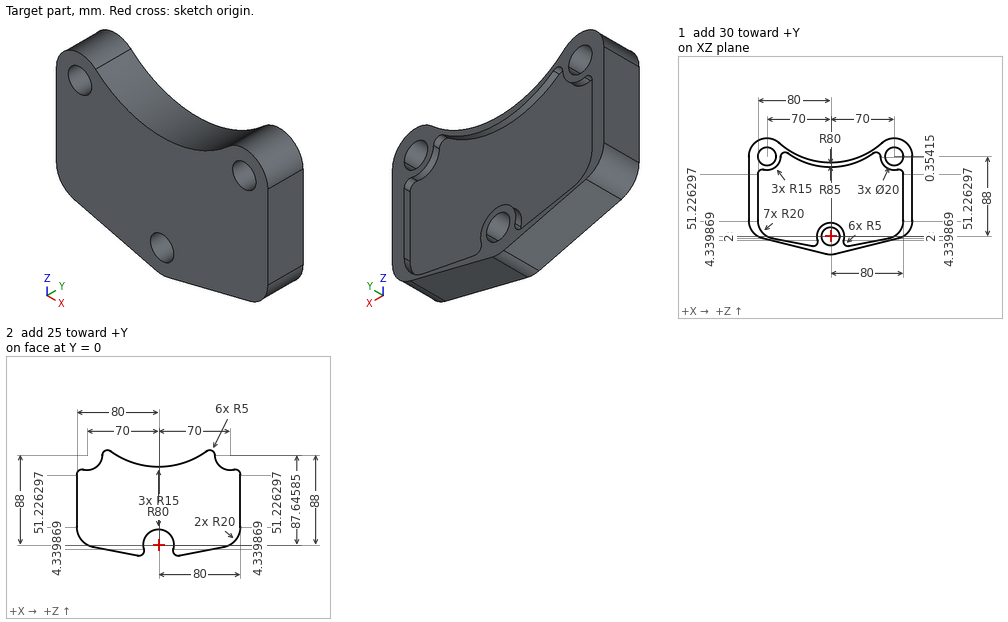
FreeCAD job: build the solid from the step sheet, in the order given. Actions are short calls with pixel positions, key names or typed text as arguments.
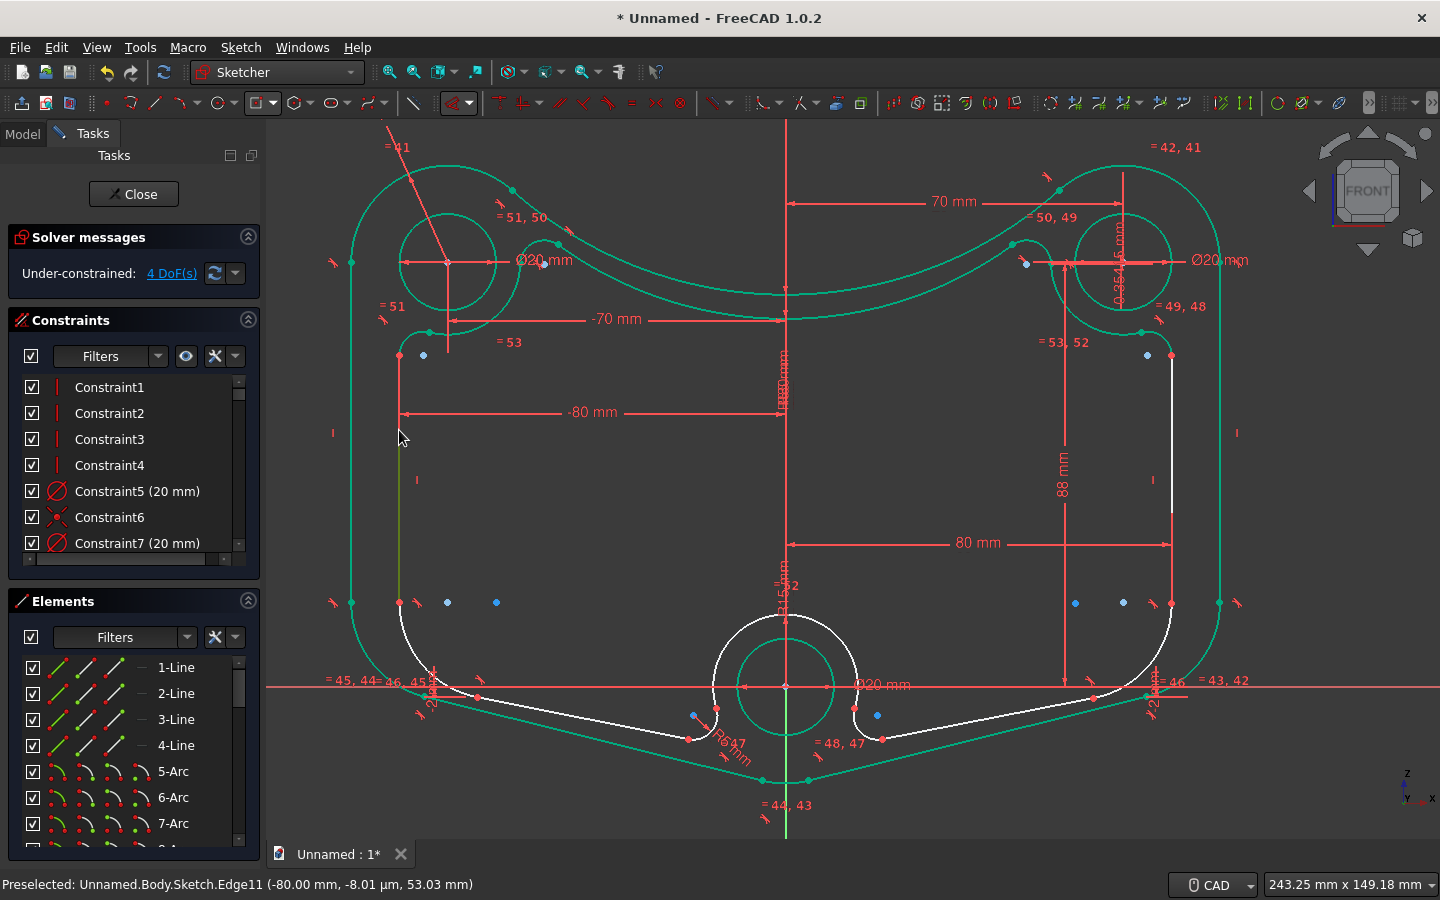
click(472, 104)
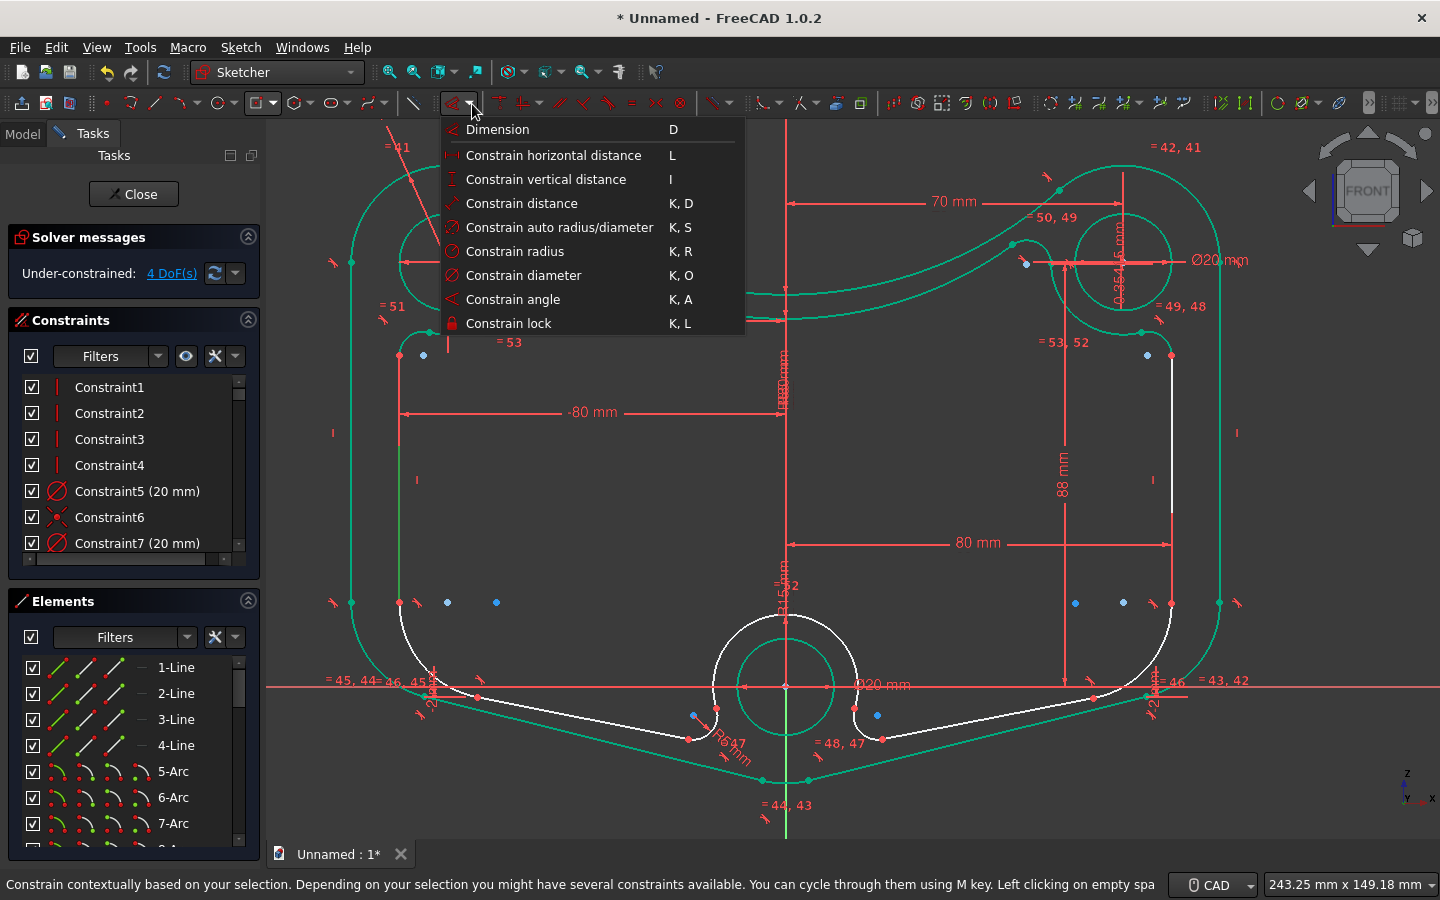
click(593, 179)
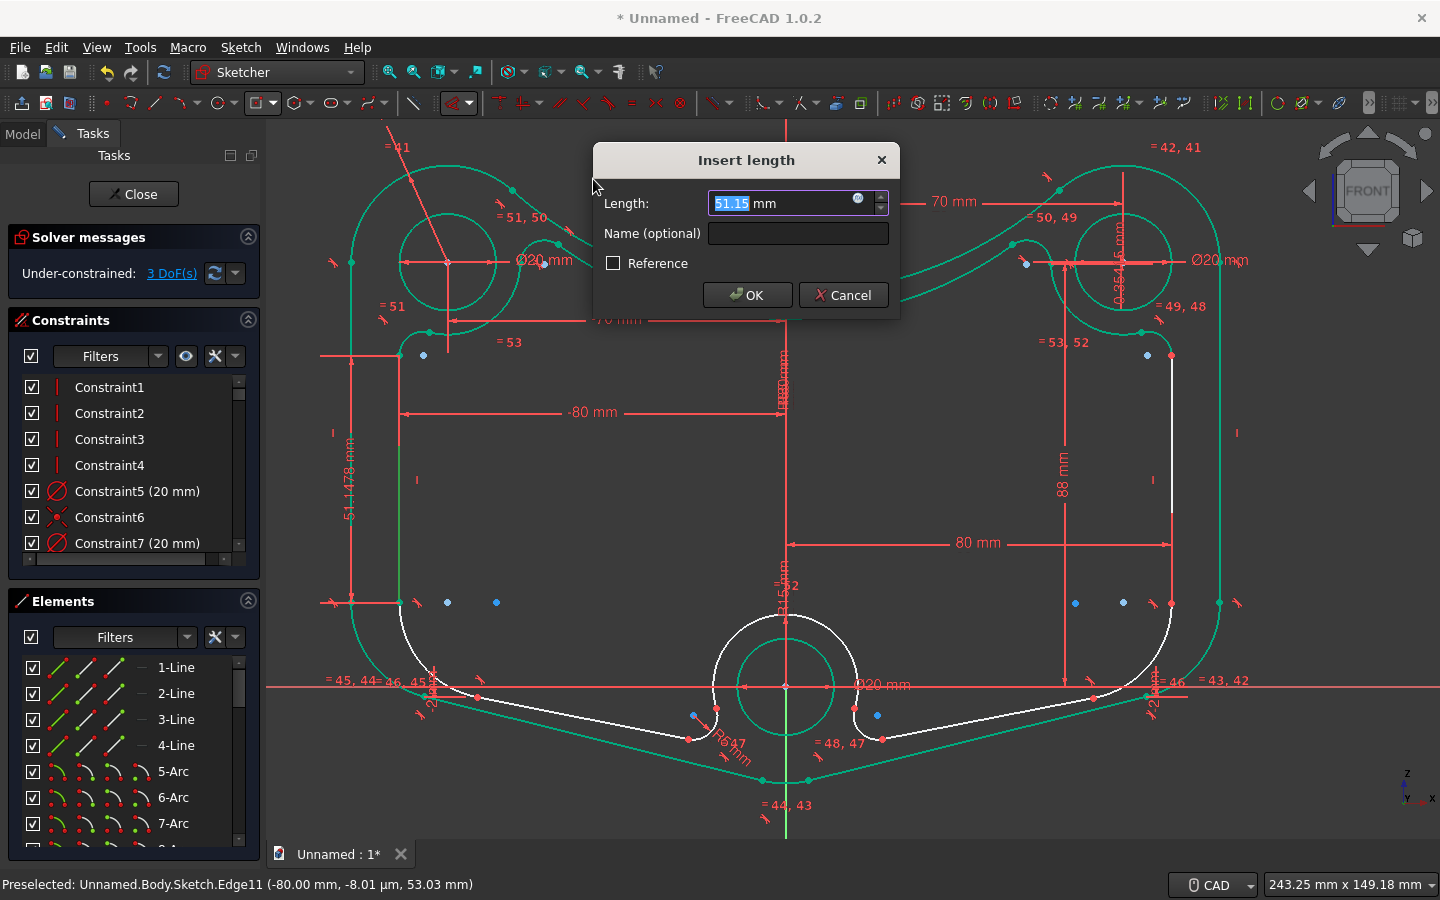
text(51.226297)
key(Return)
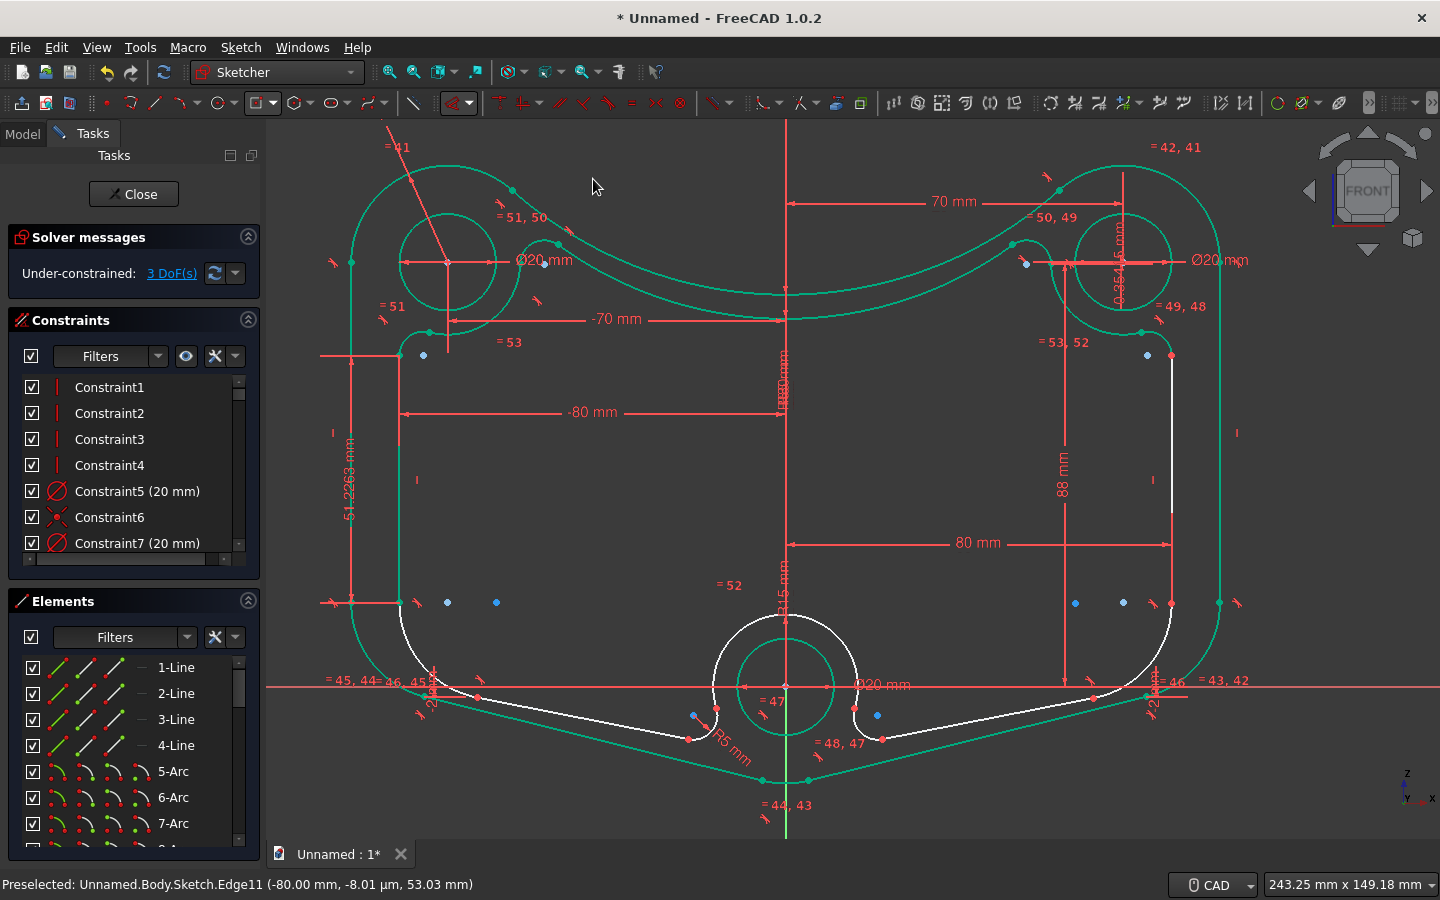
click(1172, 529)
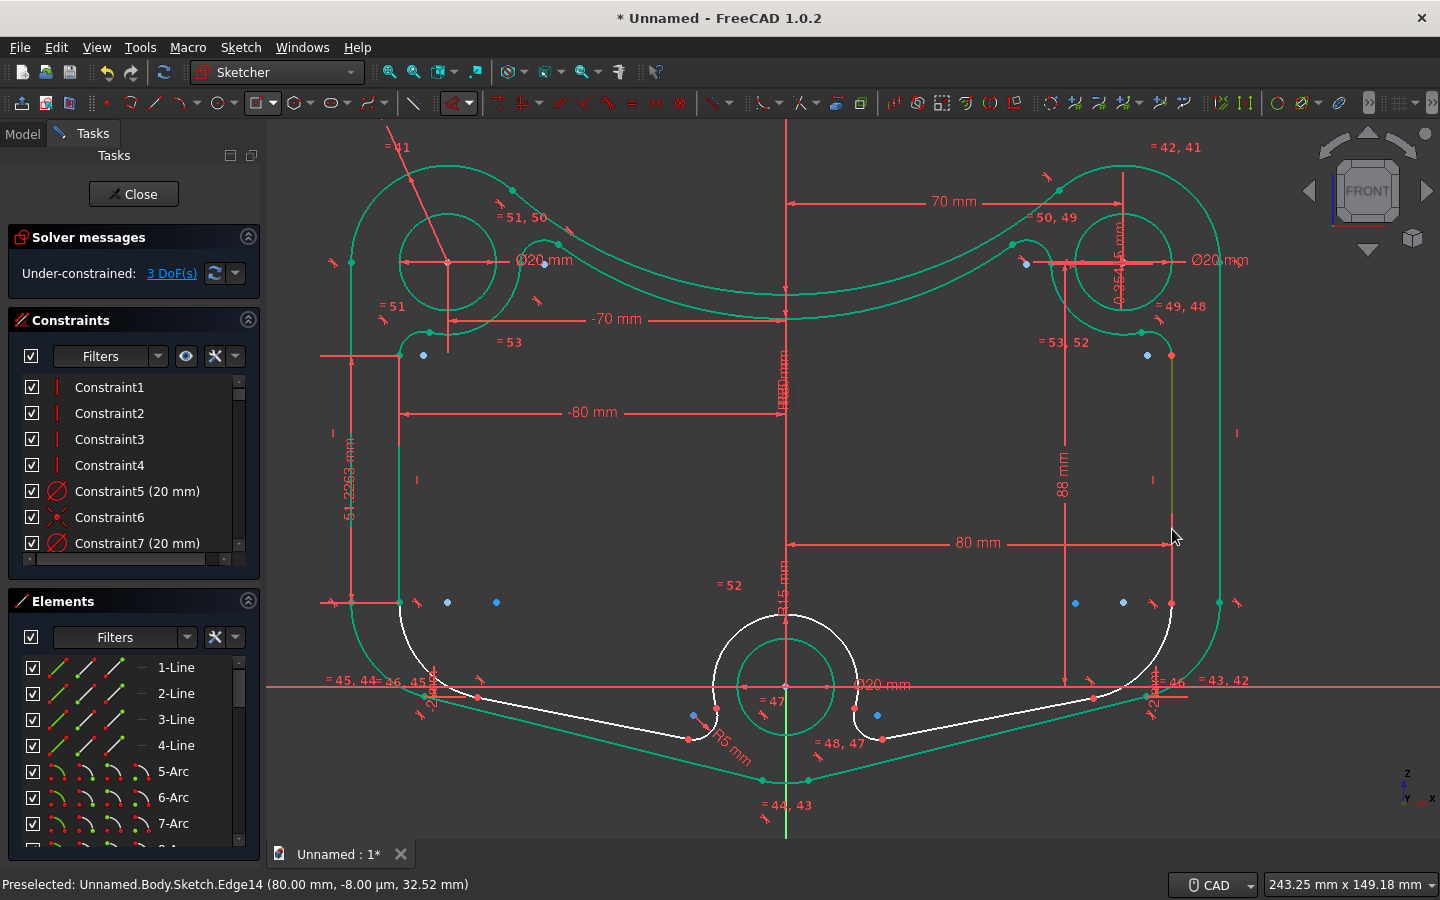
key(i)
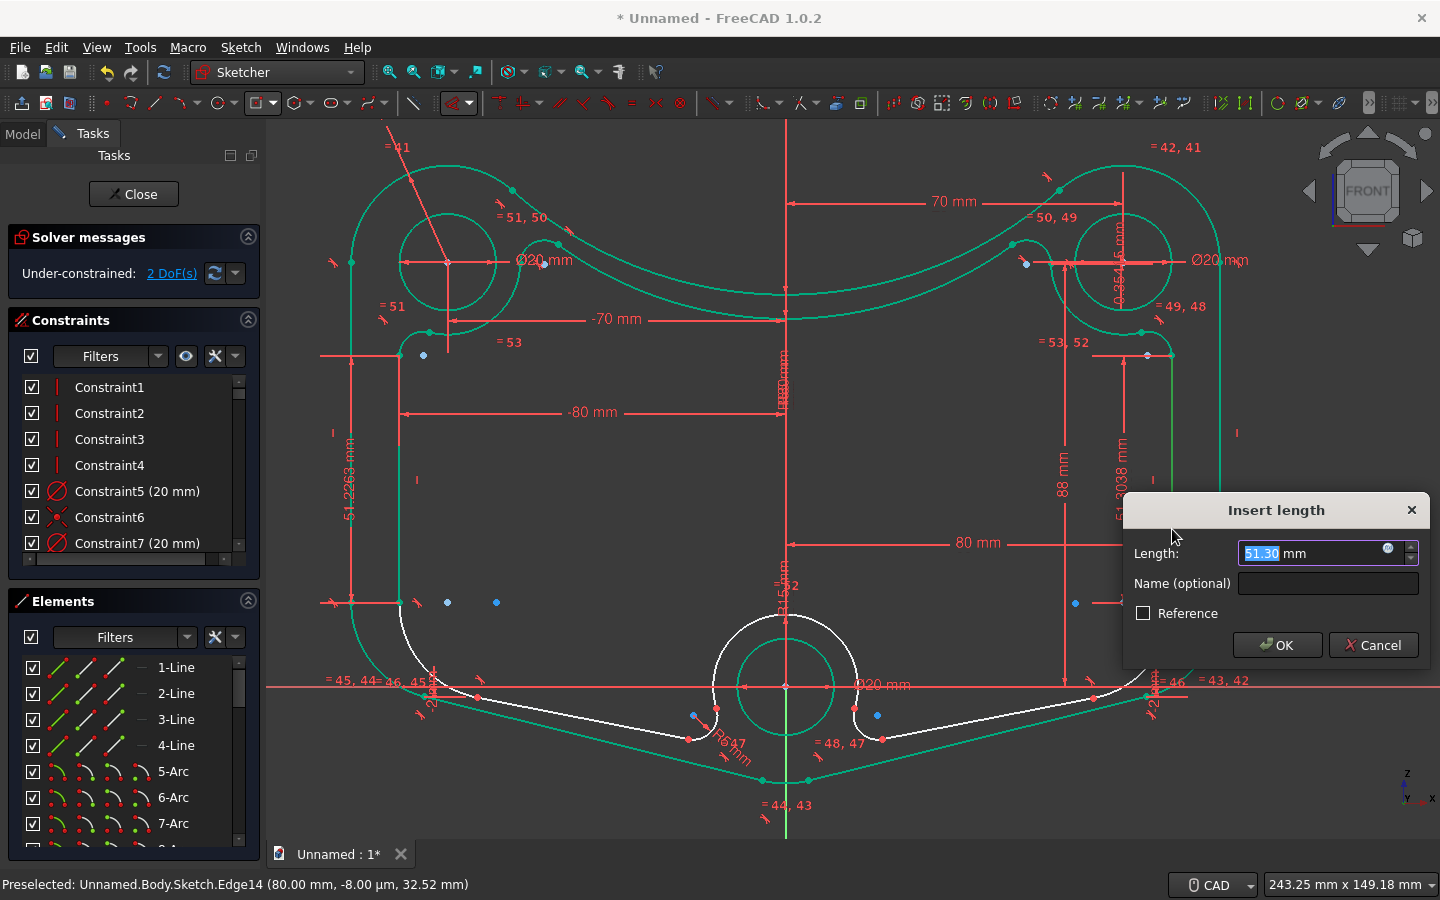
text(51.226297)
key(Return)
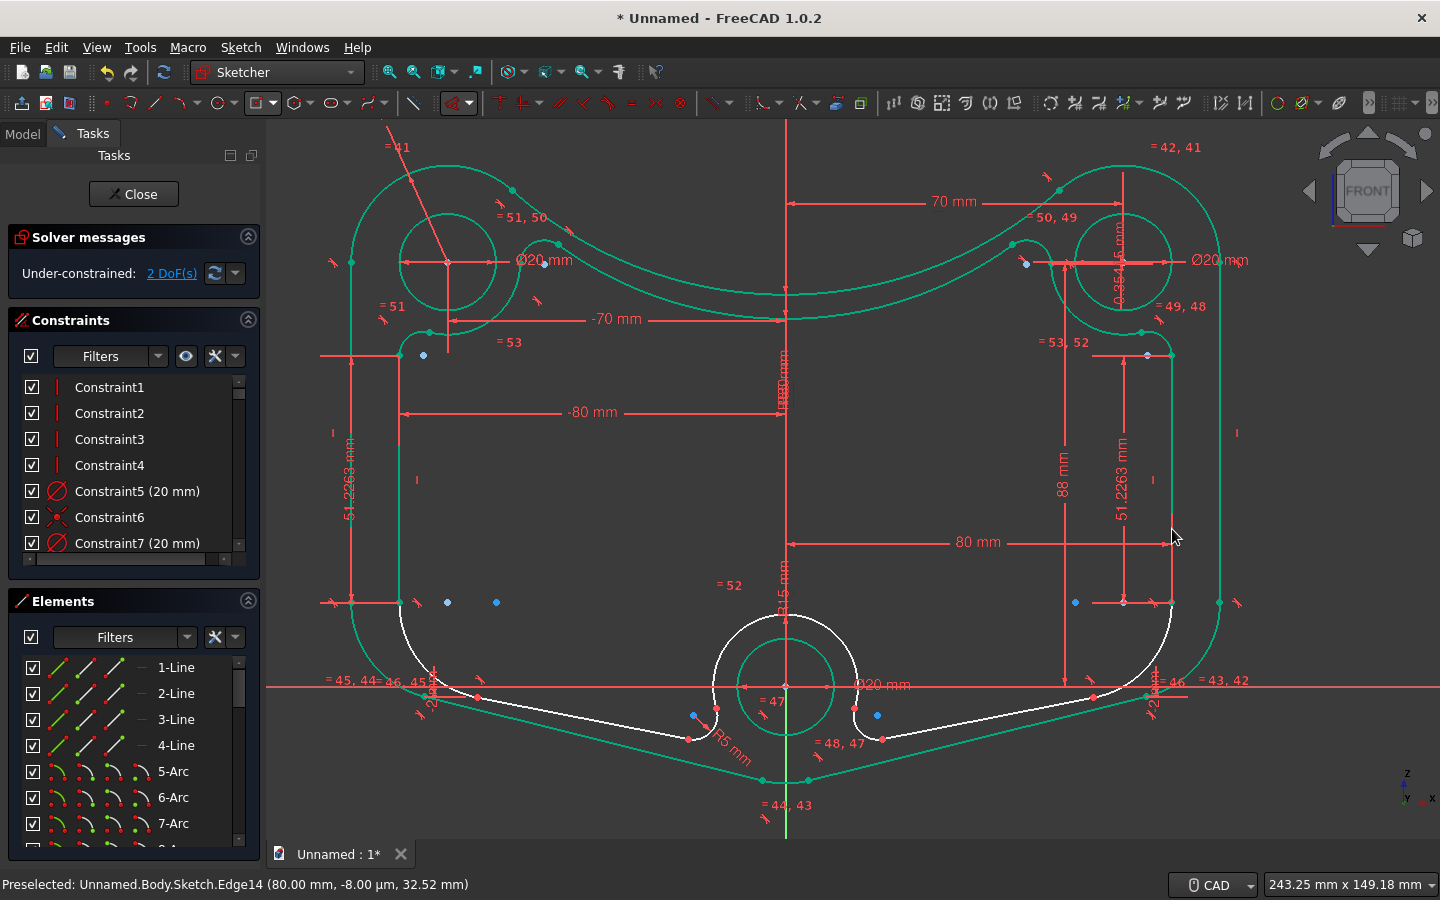
scroll(716, 708, up, 4)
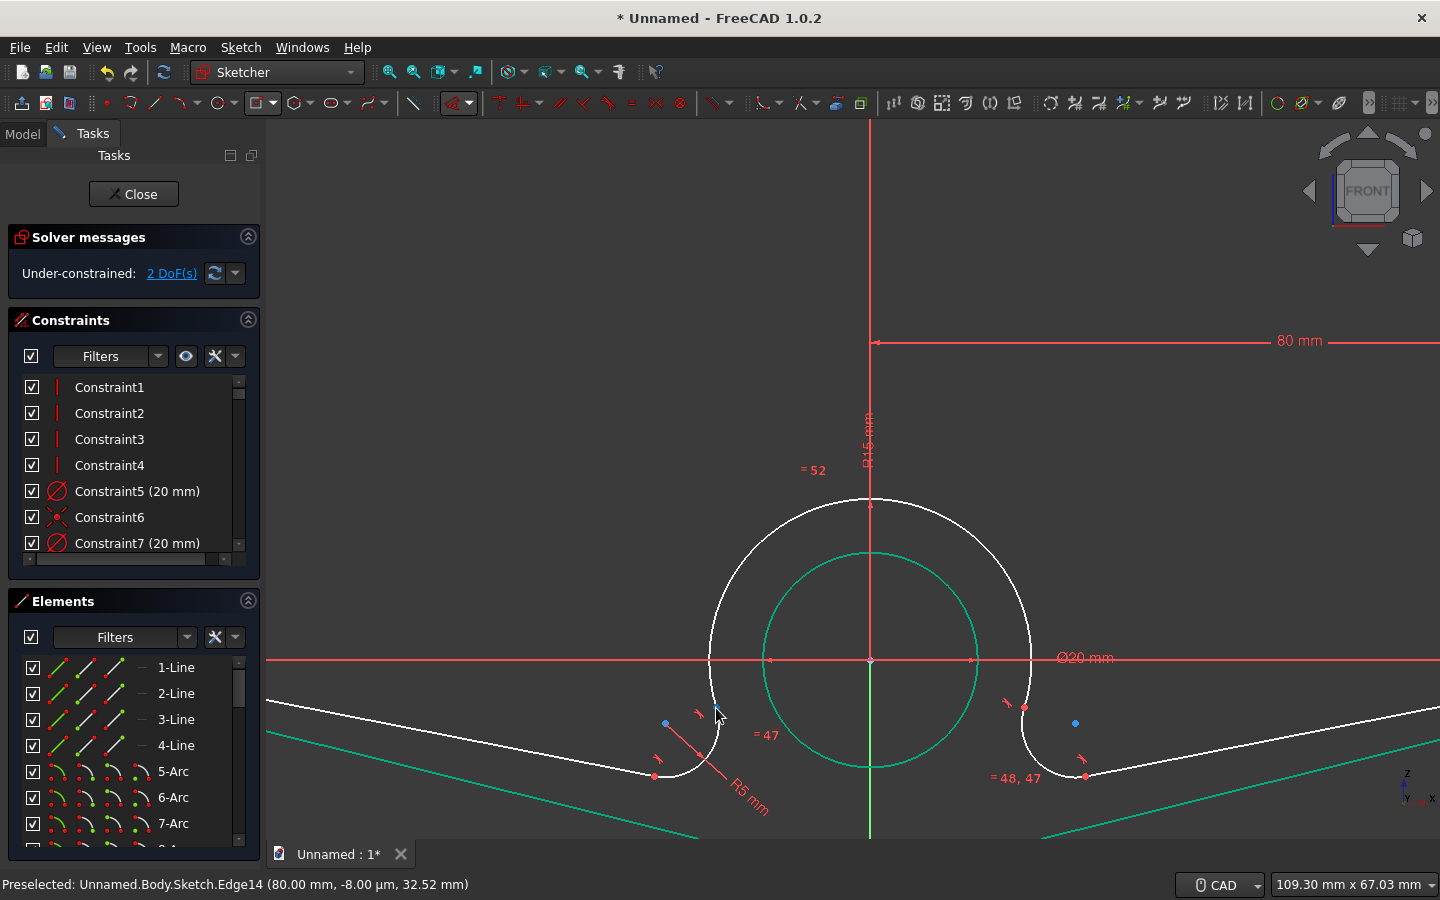
click(716, 708)